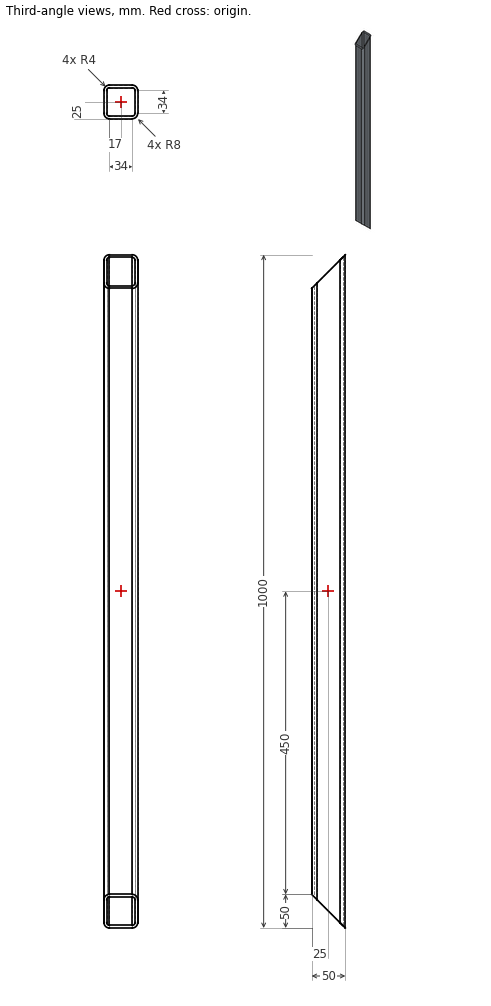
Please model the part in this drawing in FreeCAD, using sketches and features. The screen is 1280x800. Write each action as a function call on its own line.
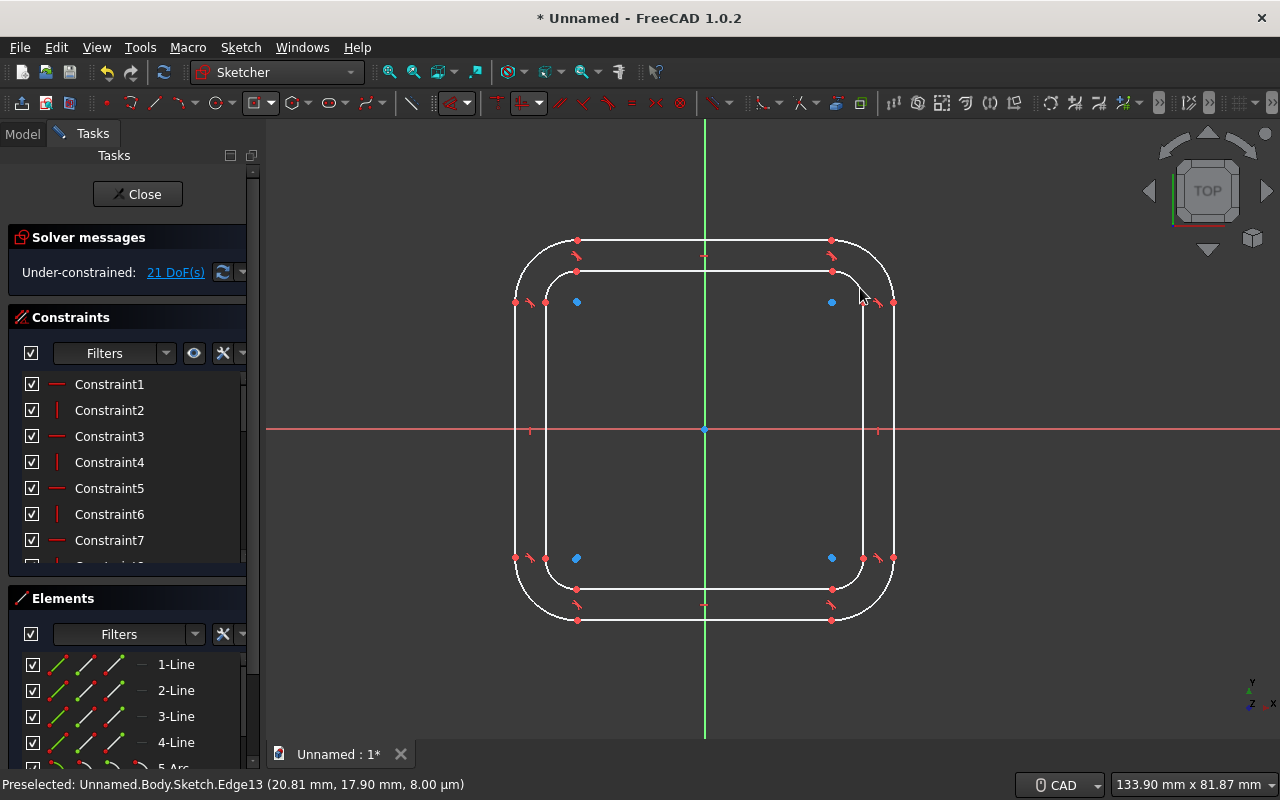
click(863, 379)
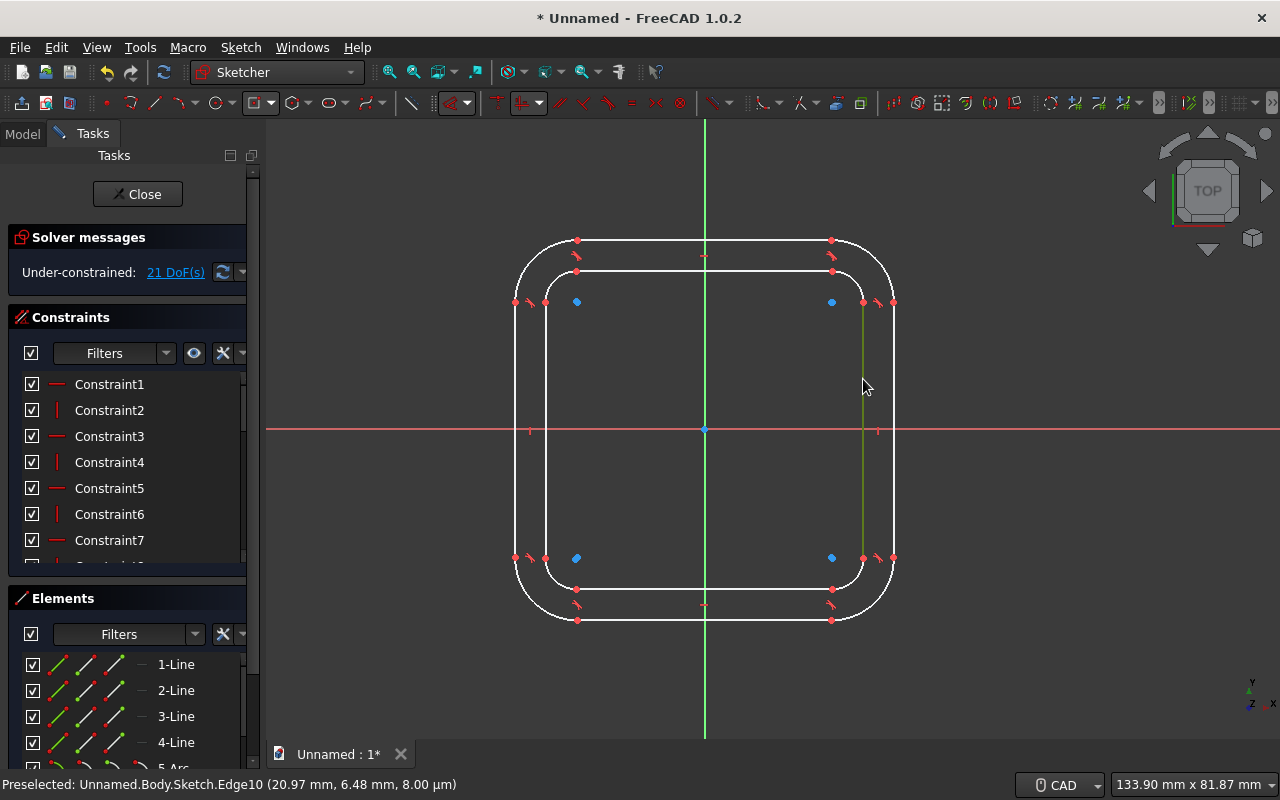
click(847, 586)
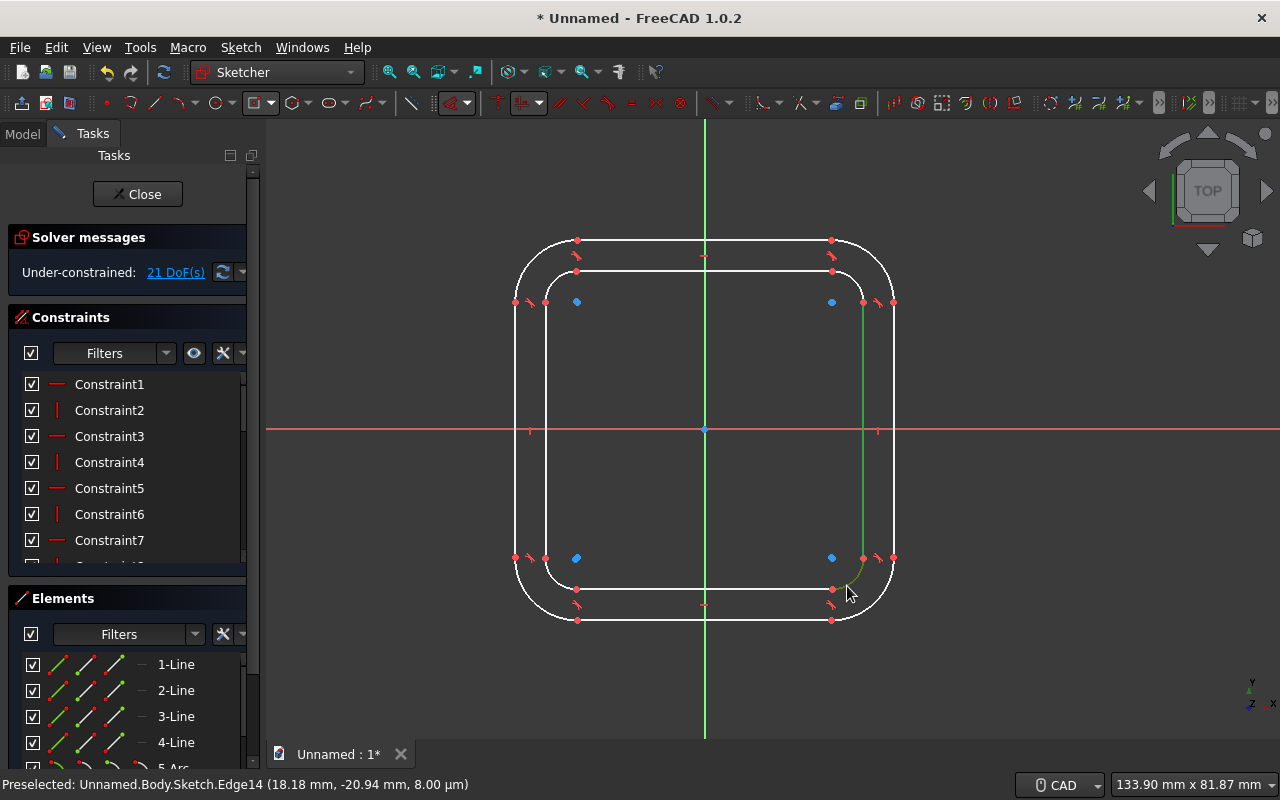
key(t)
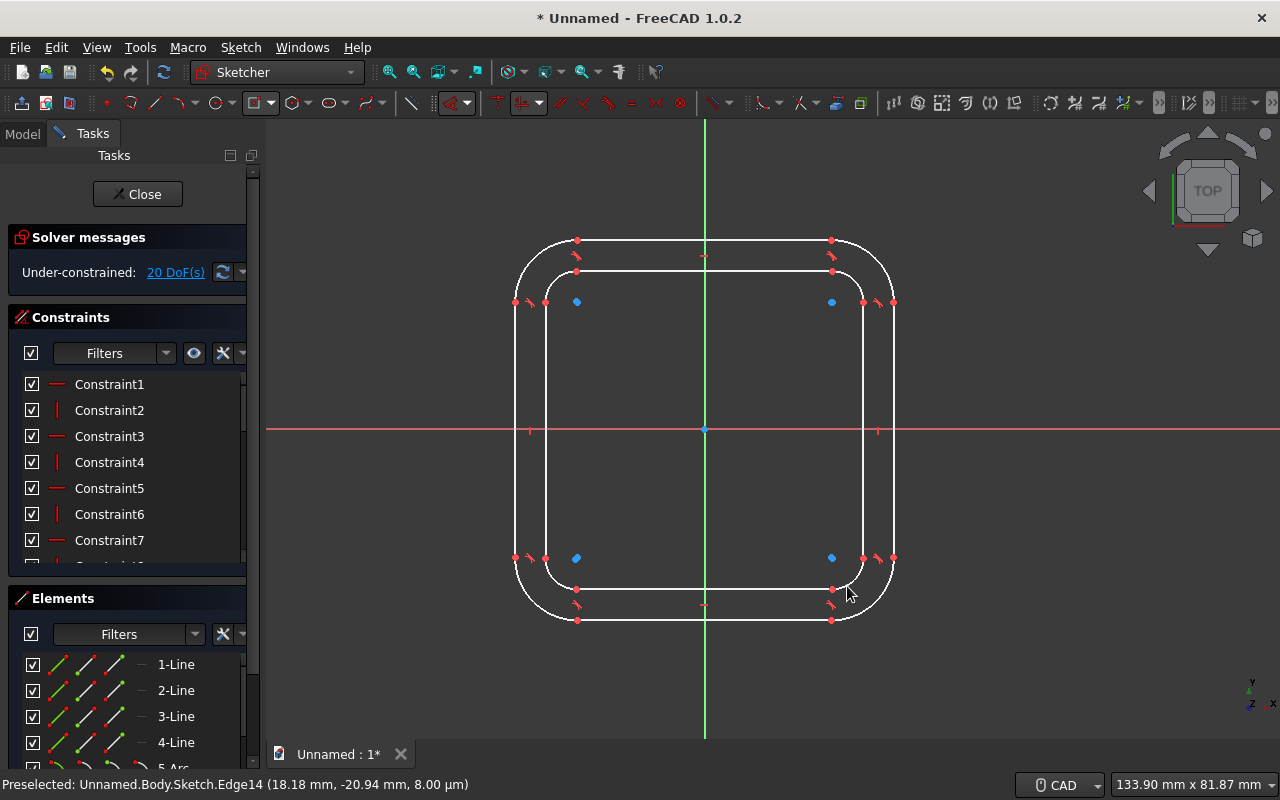
click(756, 589)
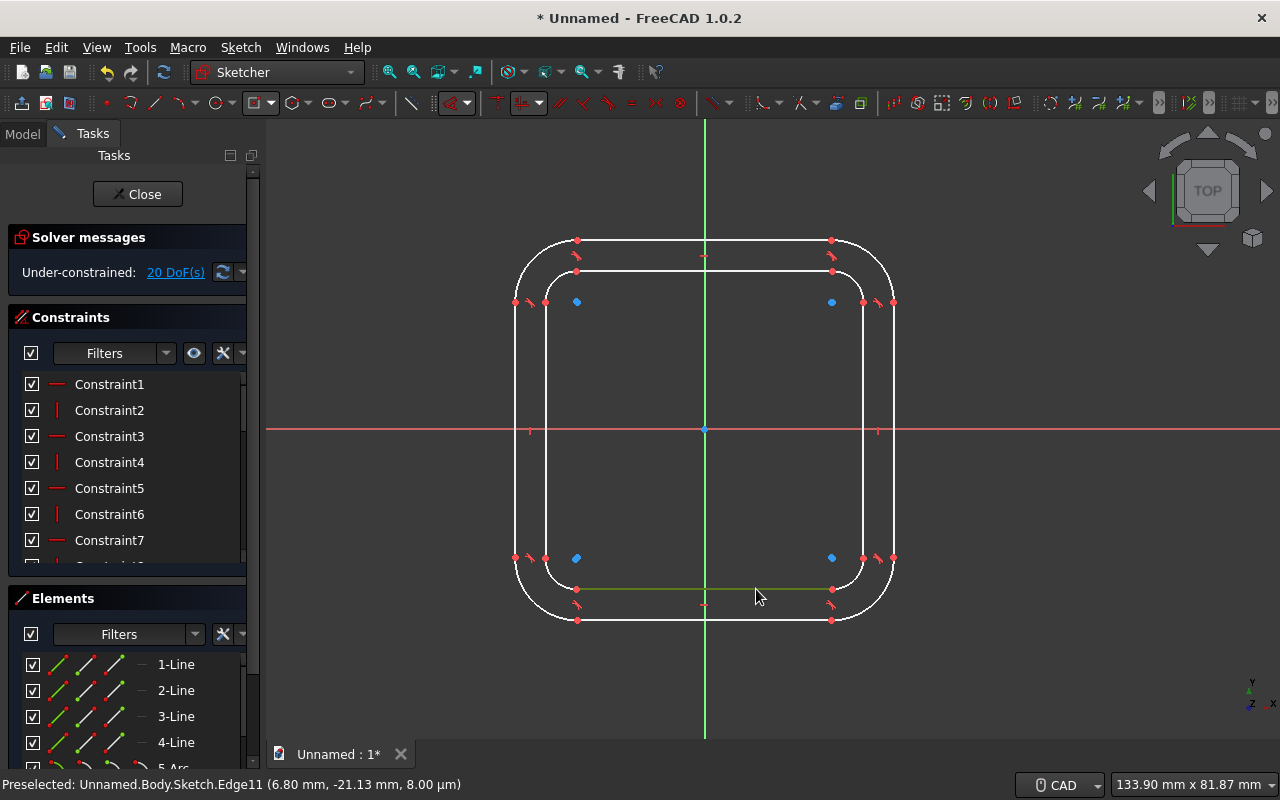
click(847, 586)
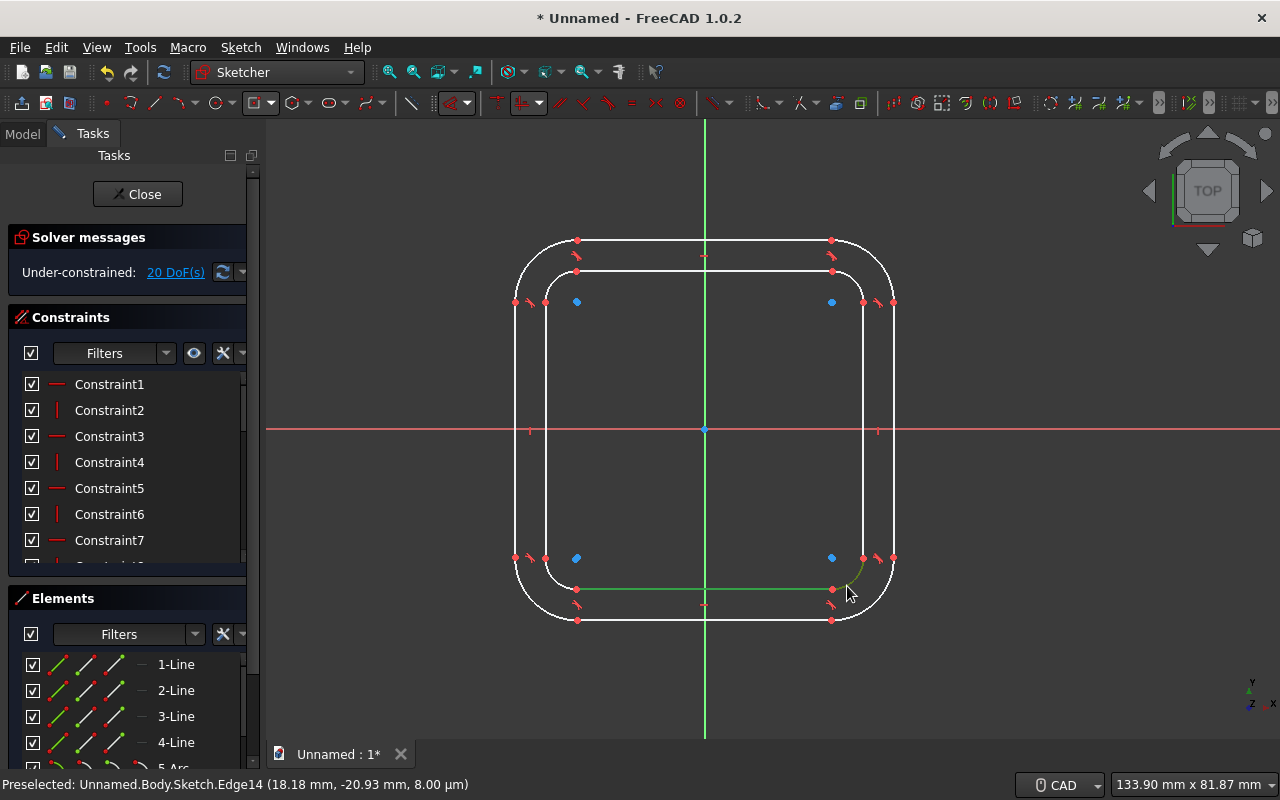
key(t)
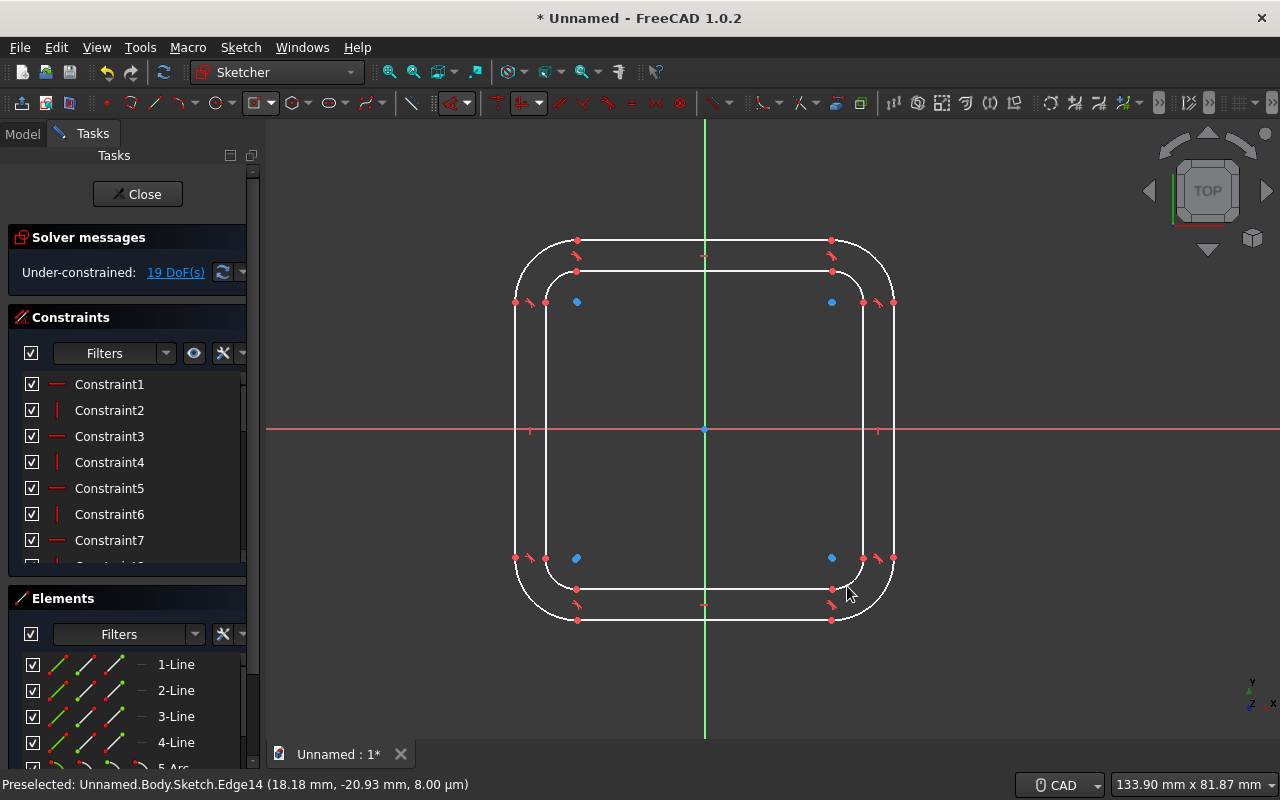
click(756, 589)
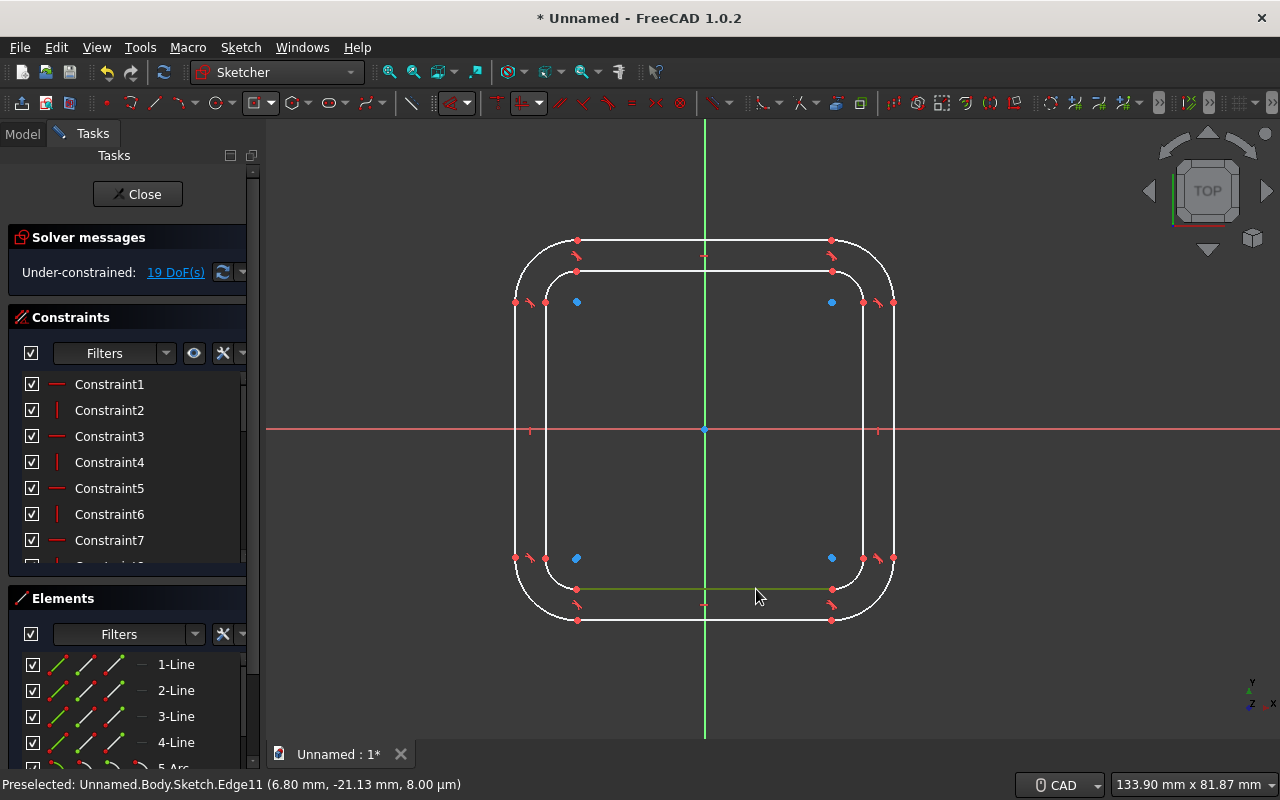
click(549, 572)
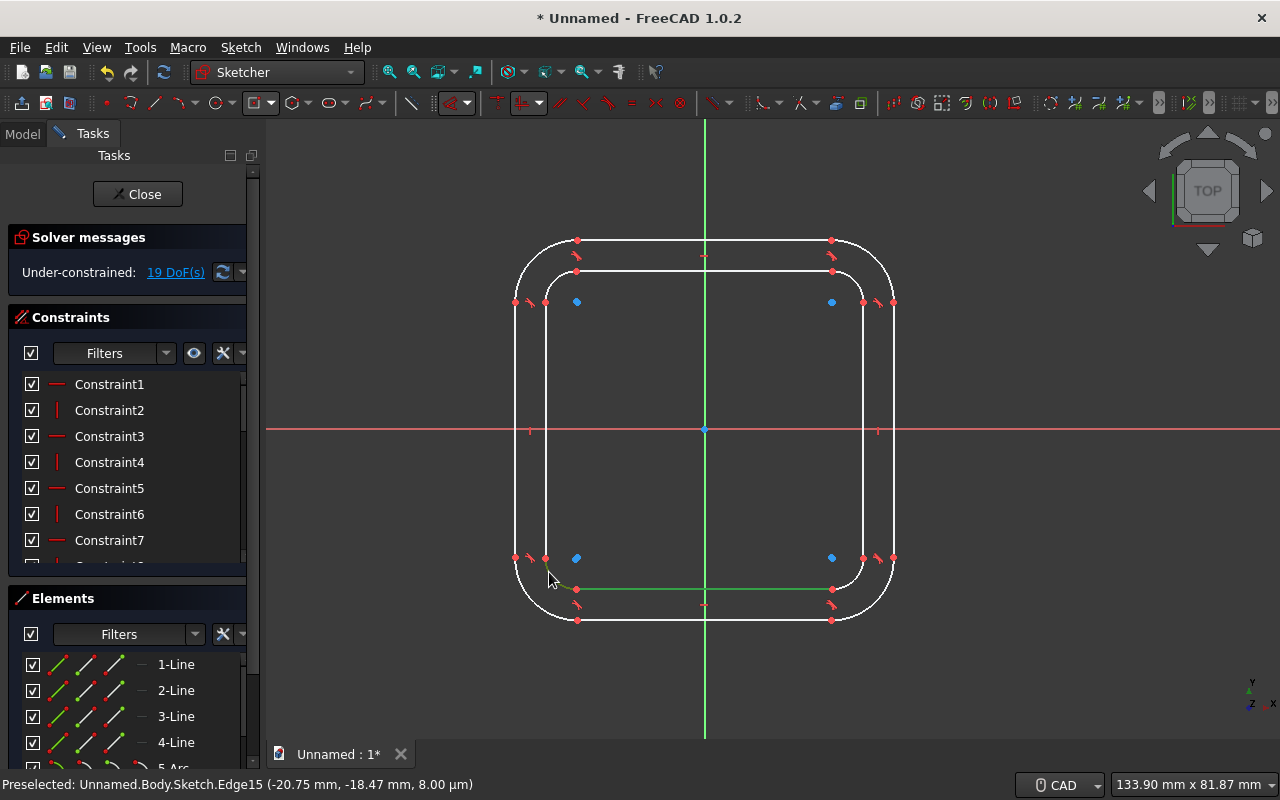
key(t)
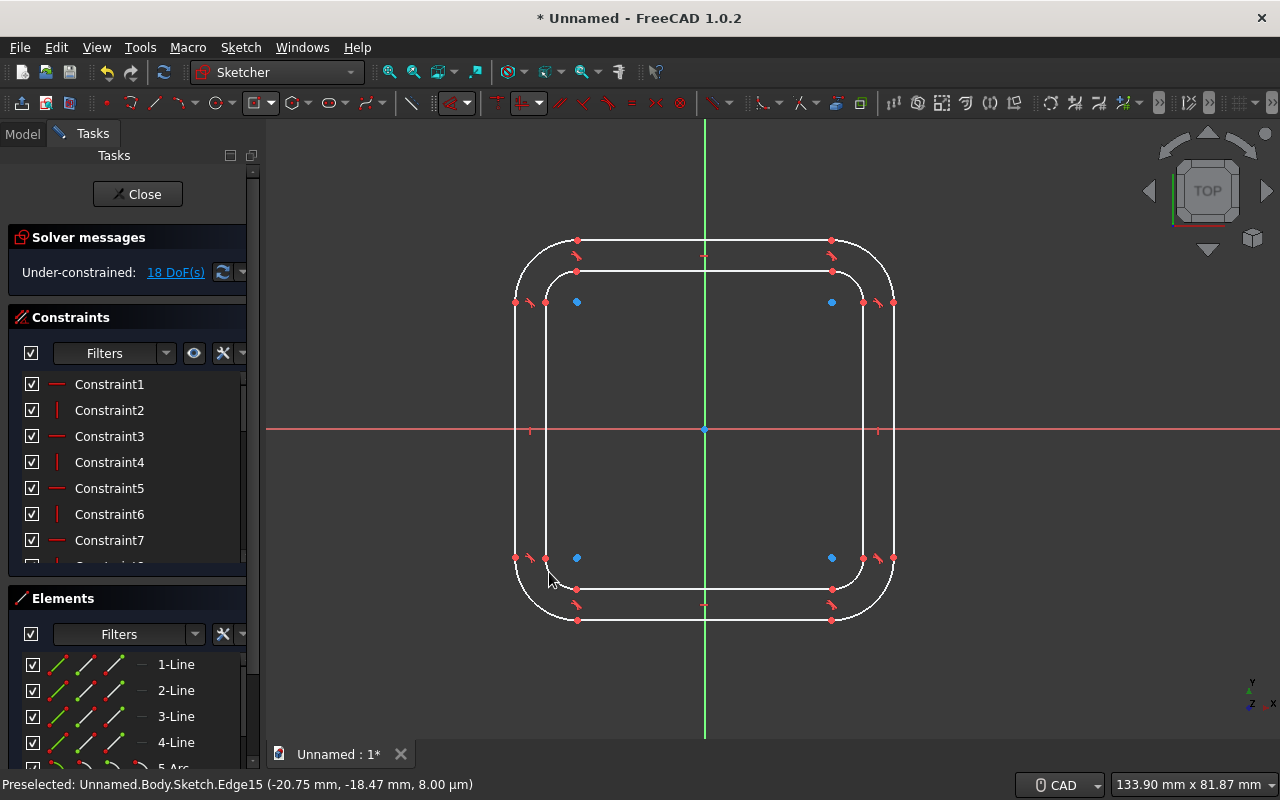
click(546, 482)